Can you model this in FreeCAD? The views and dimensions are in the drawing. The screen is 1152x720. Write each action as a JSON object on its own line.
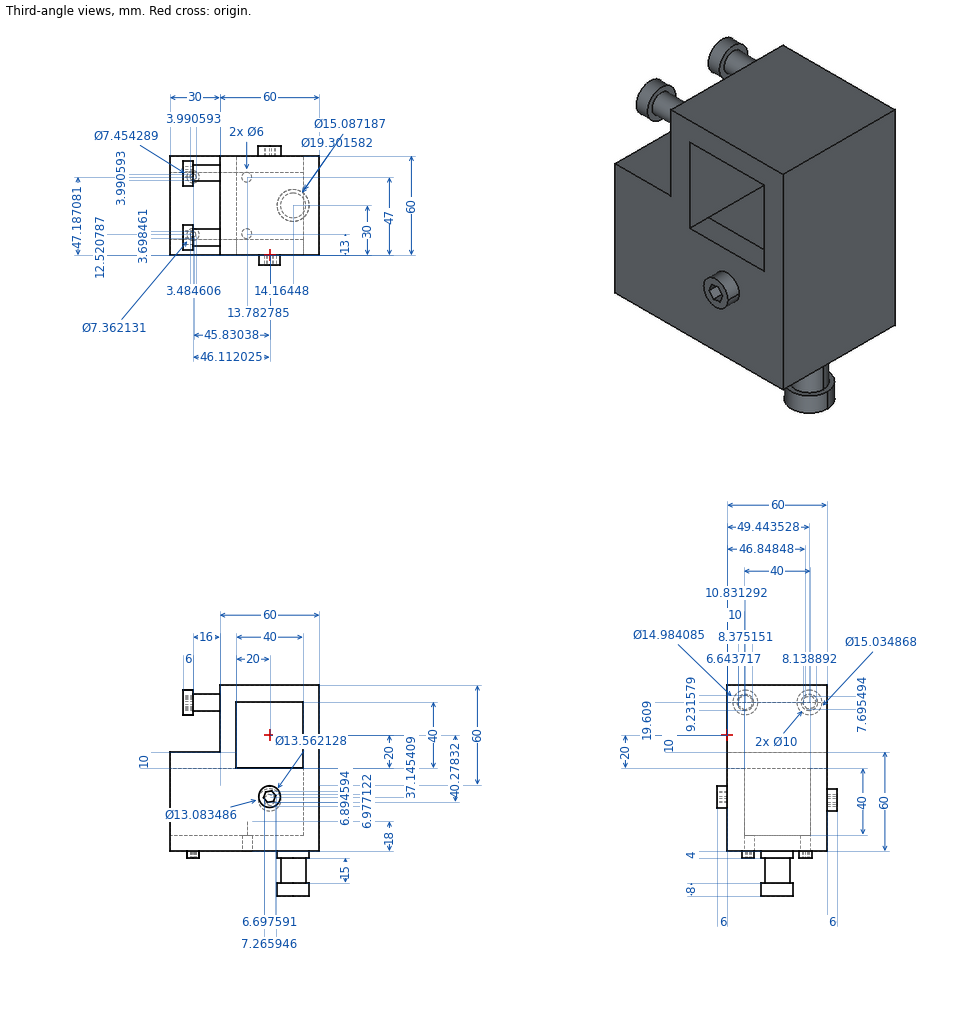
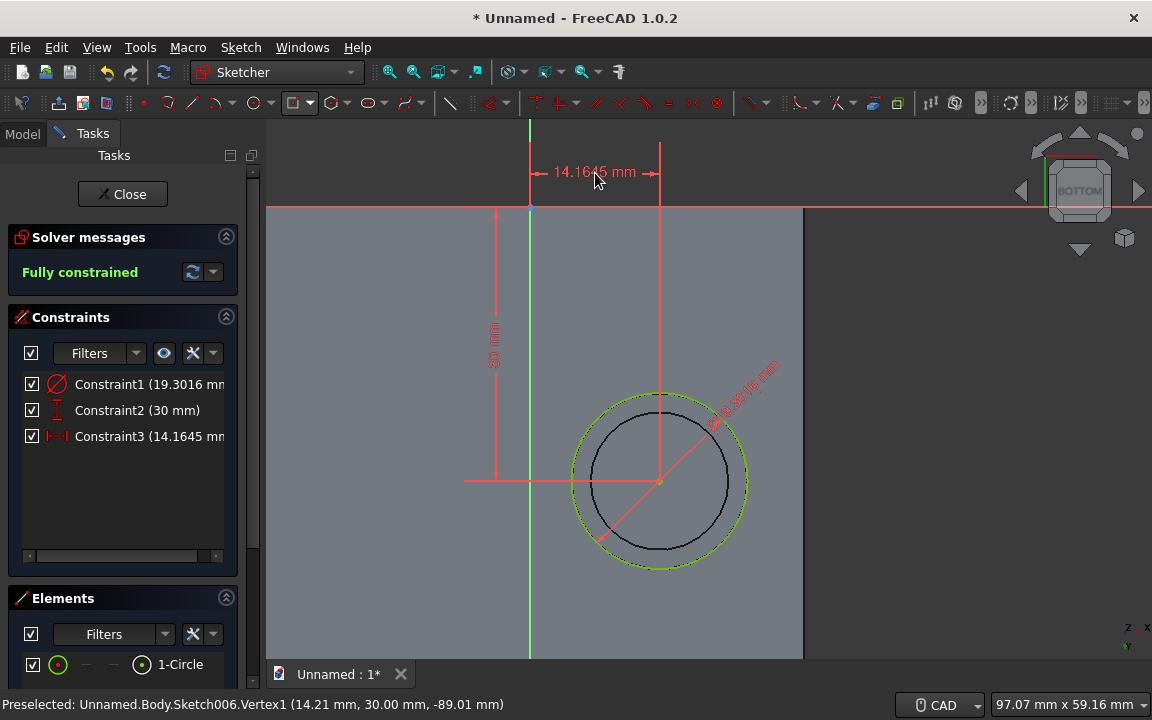
{"action": "left_click", "coordinate": [123, 194]}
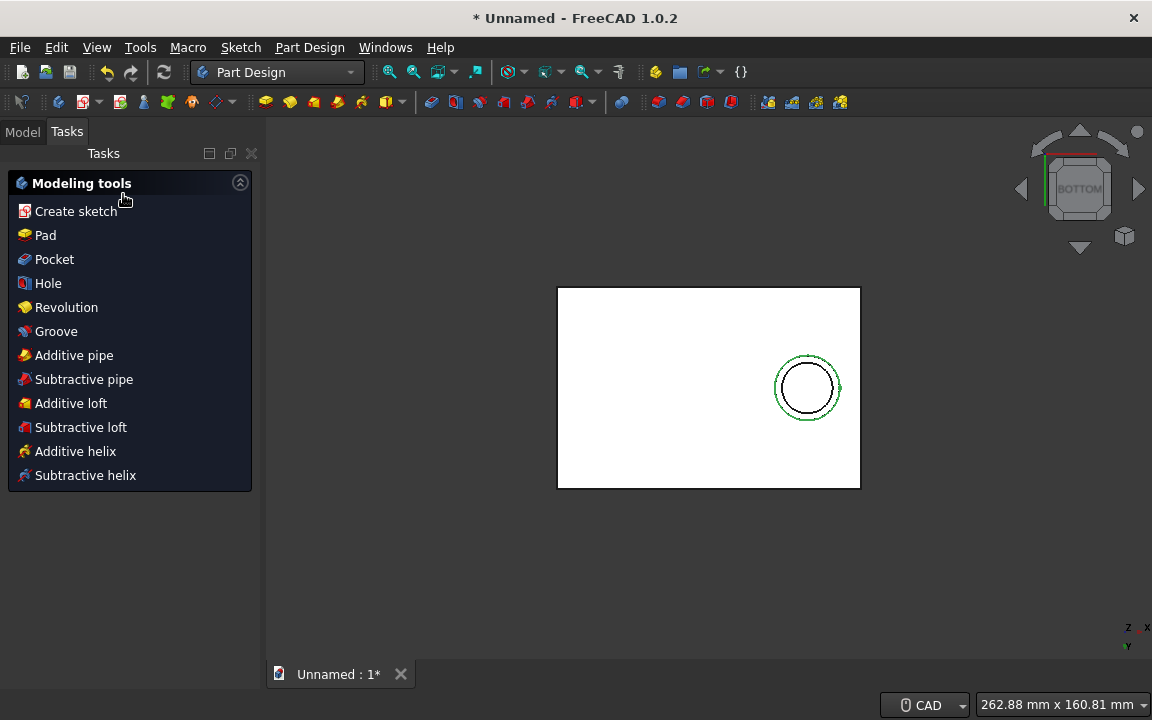
{"action": "left_click", "coordinate": [266, 102]}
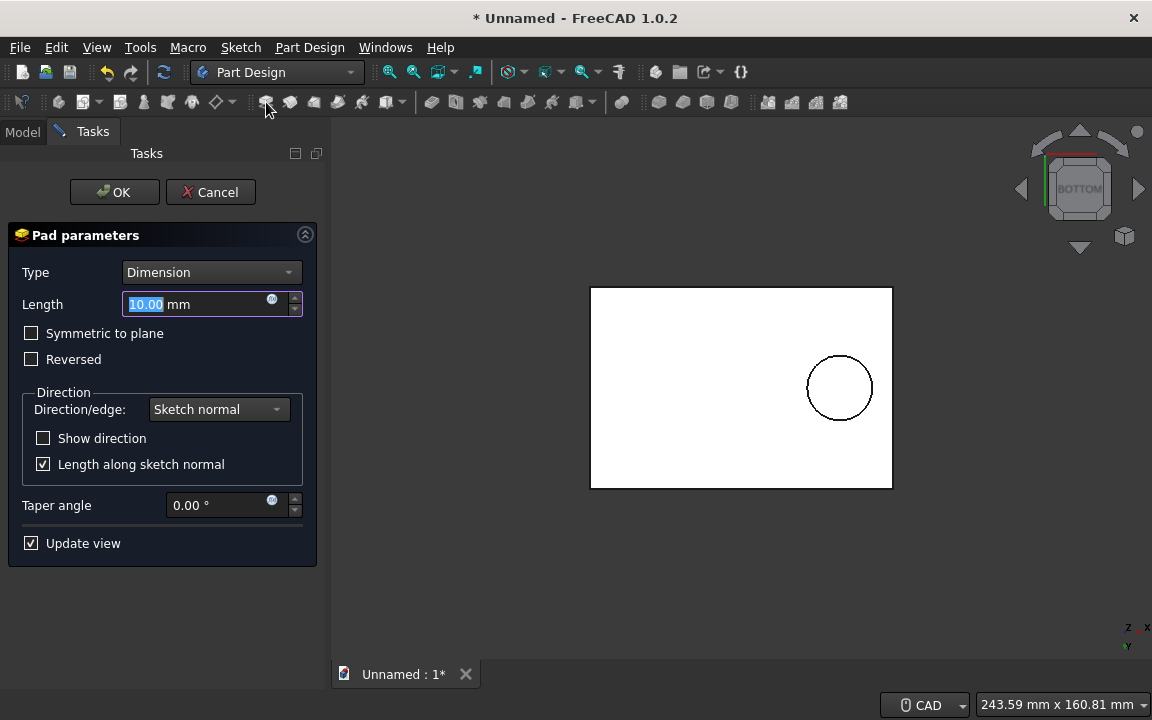
{"action": "type", "text": "8"}
{"action": "key", "text": "Tab"}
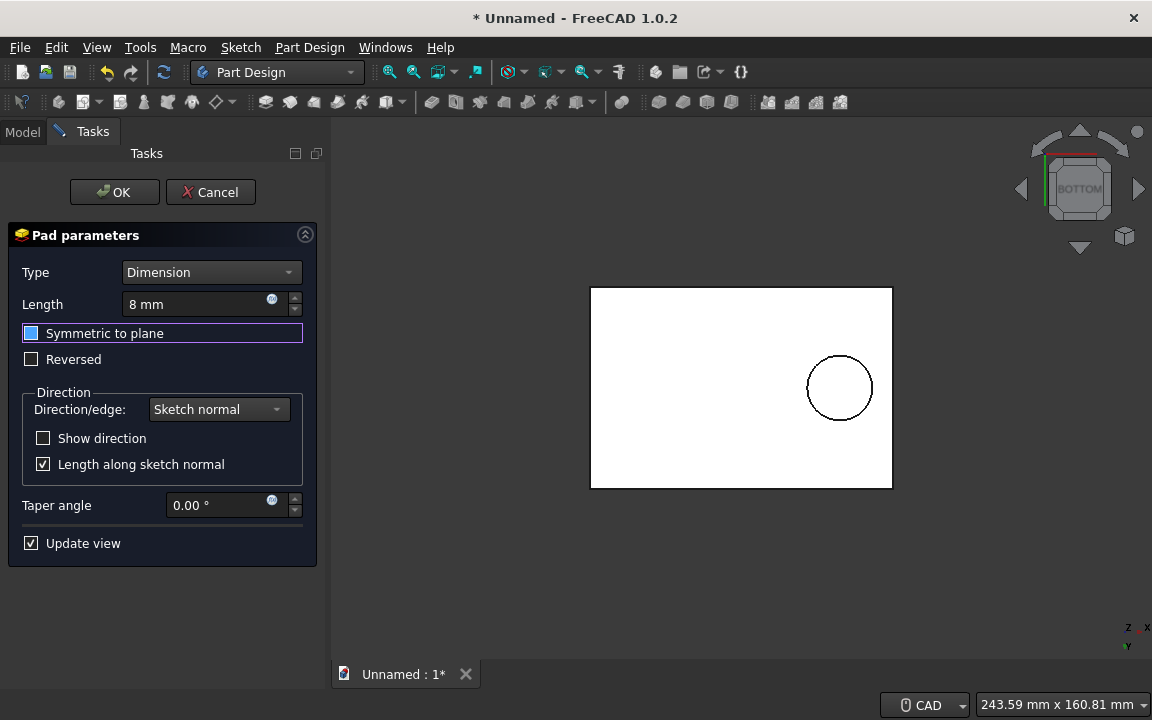
{"action": "left_click", "coordinate": [115, 192]}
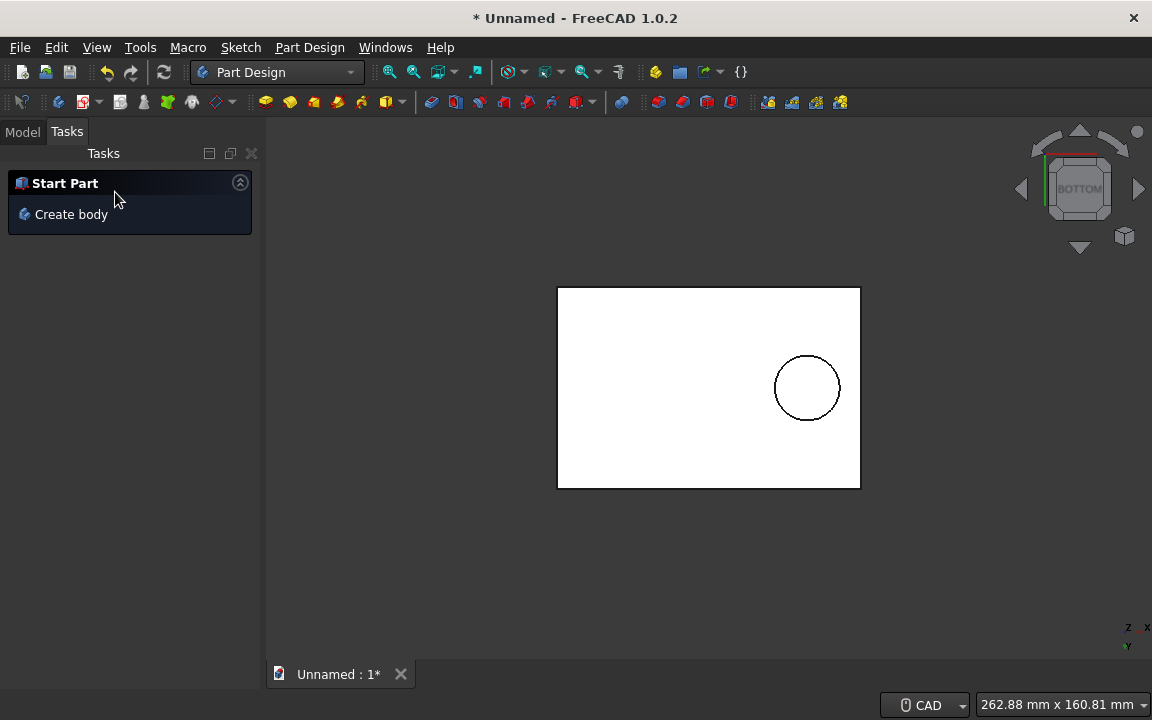
{"action": "left_click", "coordinate": [390, 72]}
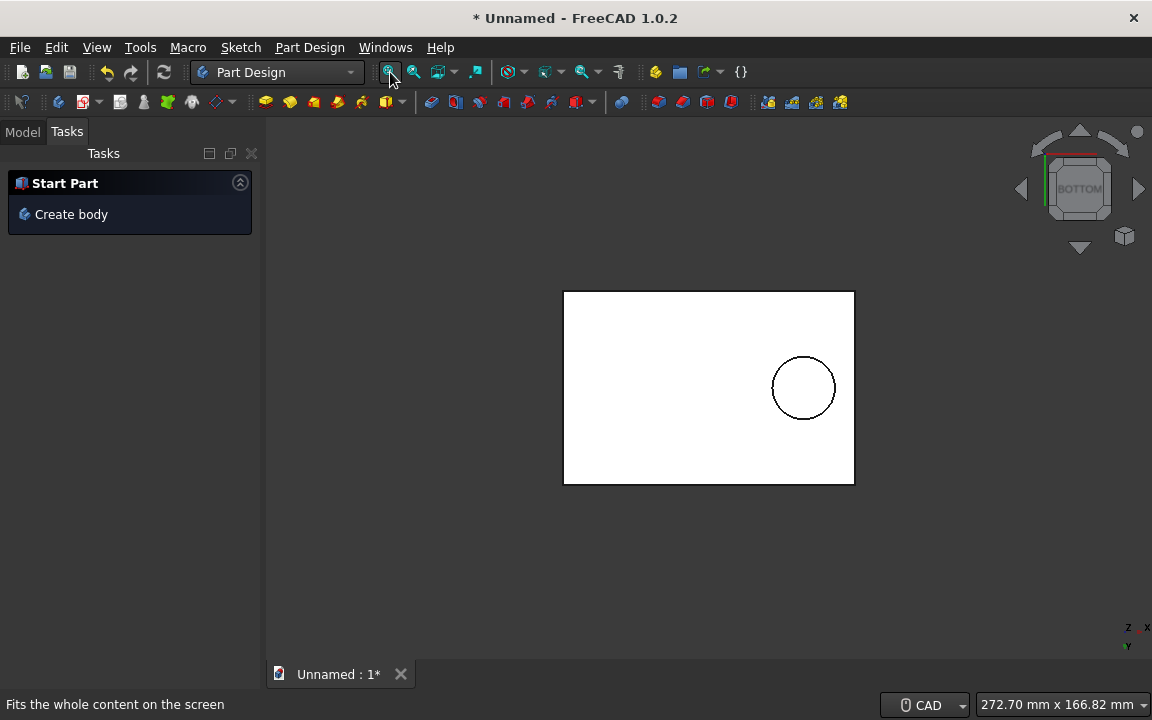
{"action": "left_click", "coordinate": [667, 387]}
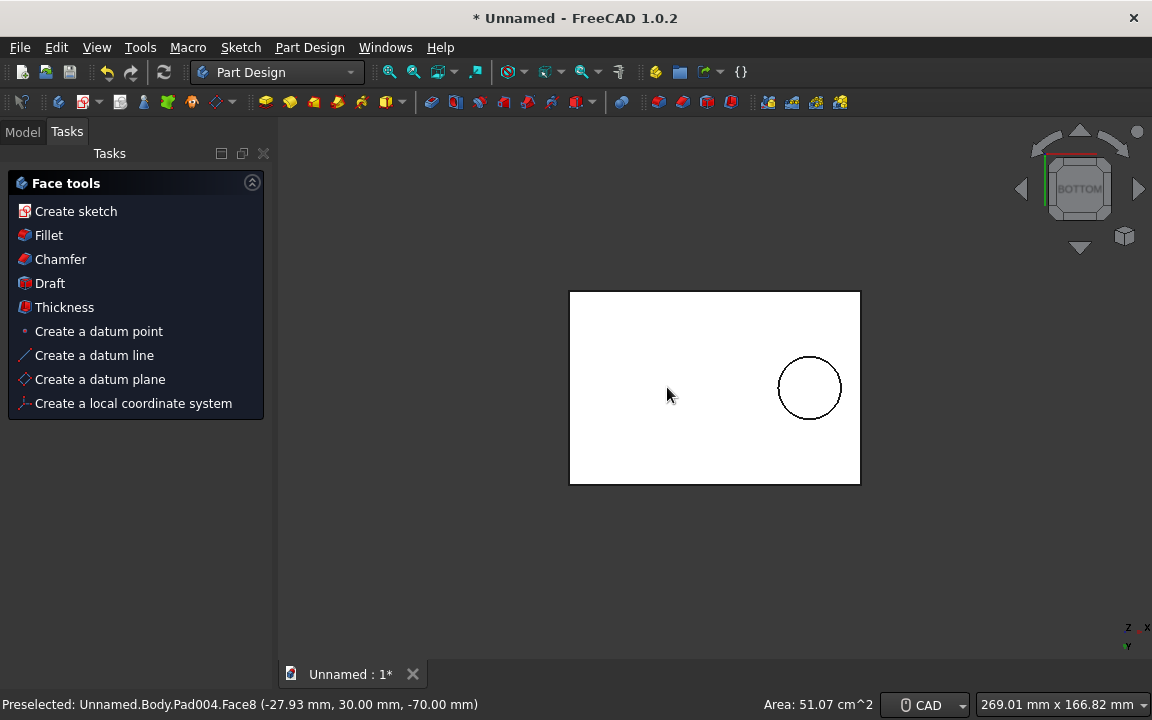
{"action": "left_click", "coordinate": [84, 102]}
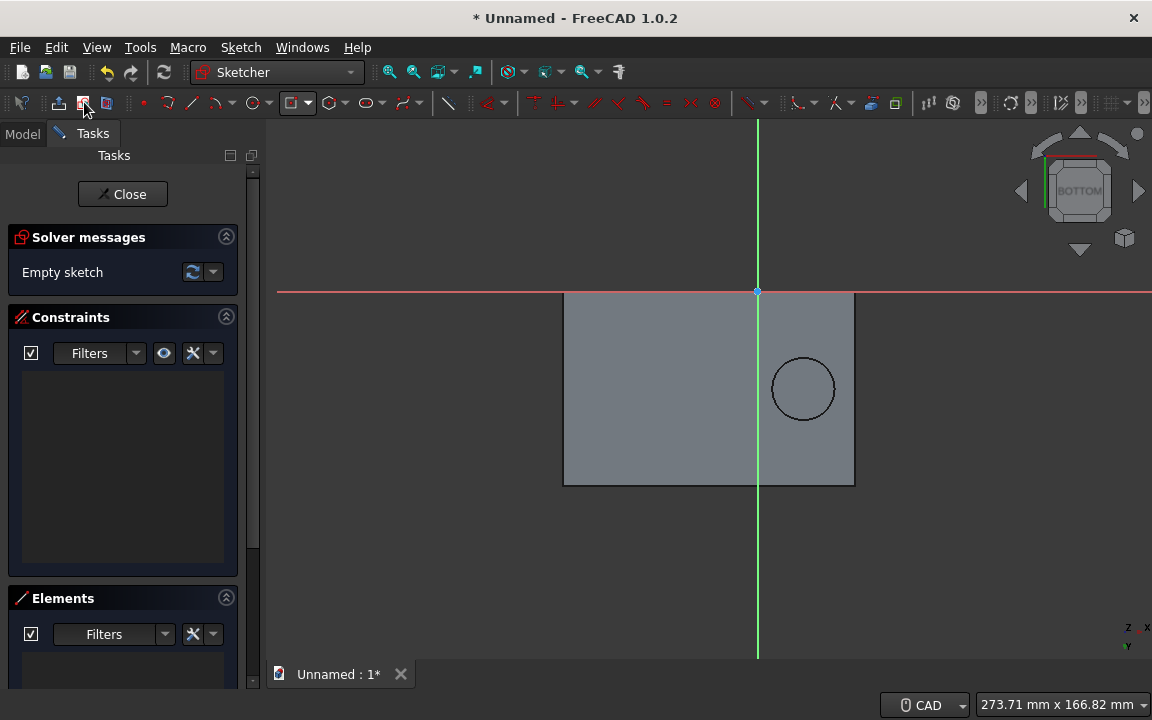
{"action": "scroll", "coordinate": [804, 360], "scroll_direction": "up", "scroll_amount": 4}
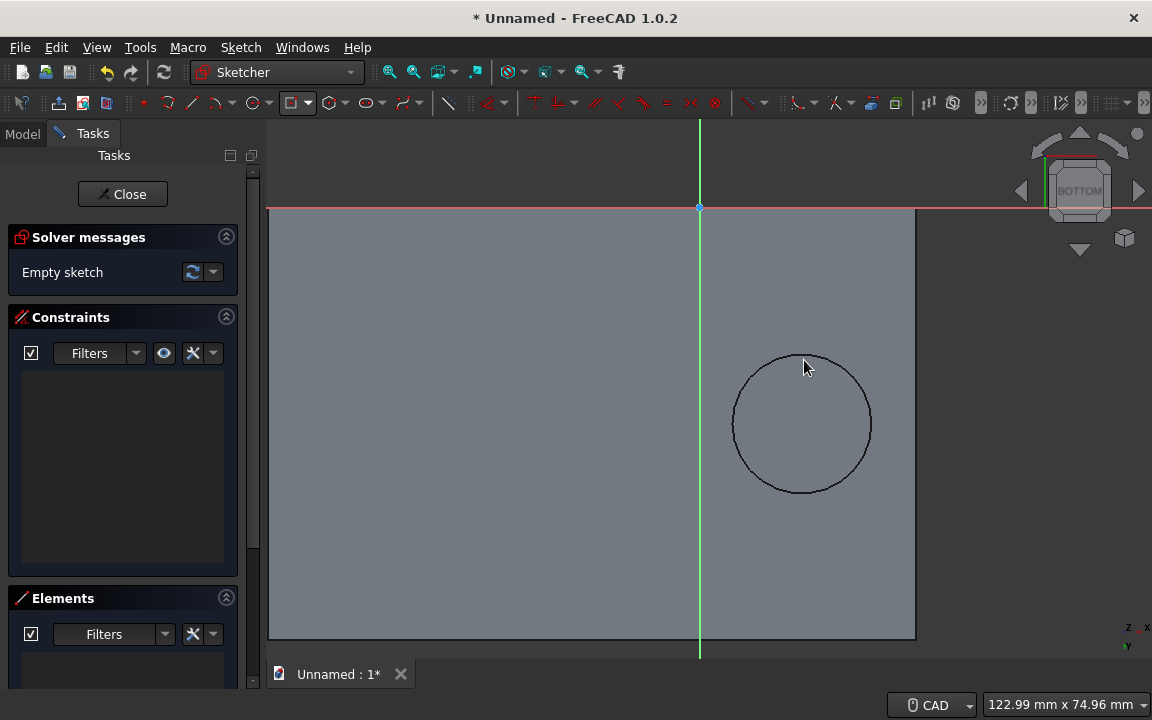
{"action": "left_click", "coordinate": [254, 104]}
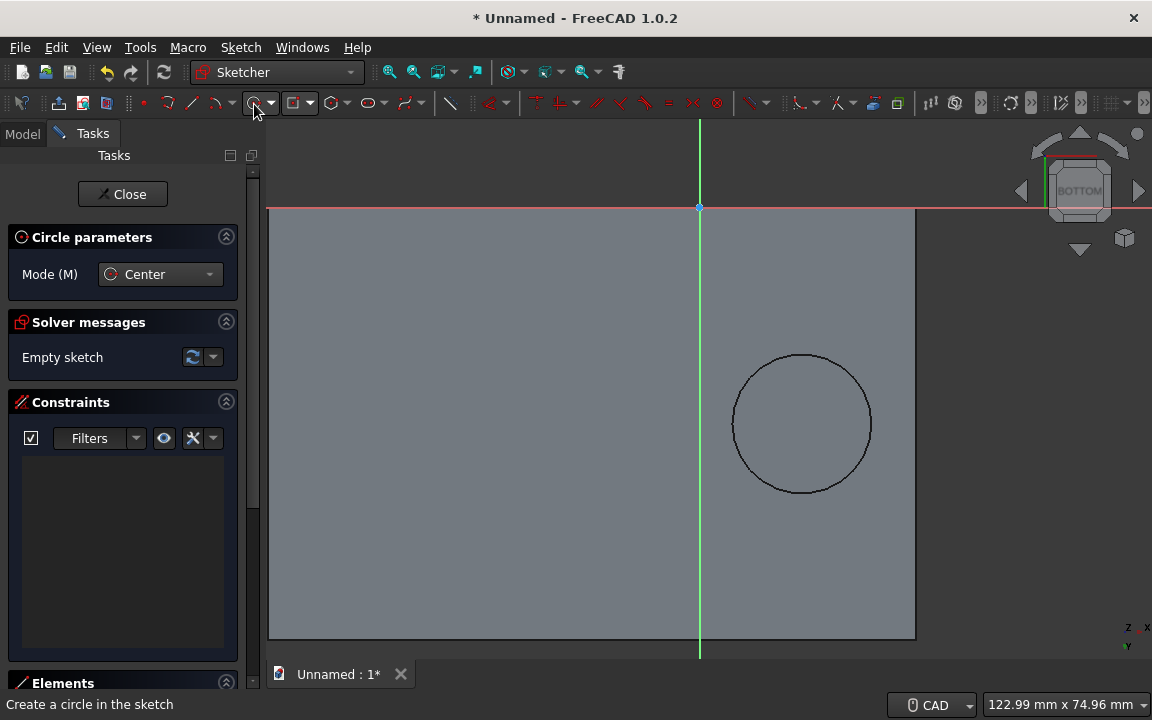
{"action": "left_click", "coordinate": [601, 546]}
{"action": "left_click", "coordinate": [616, 531]}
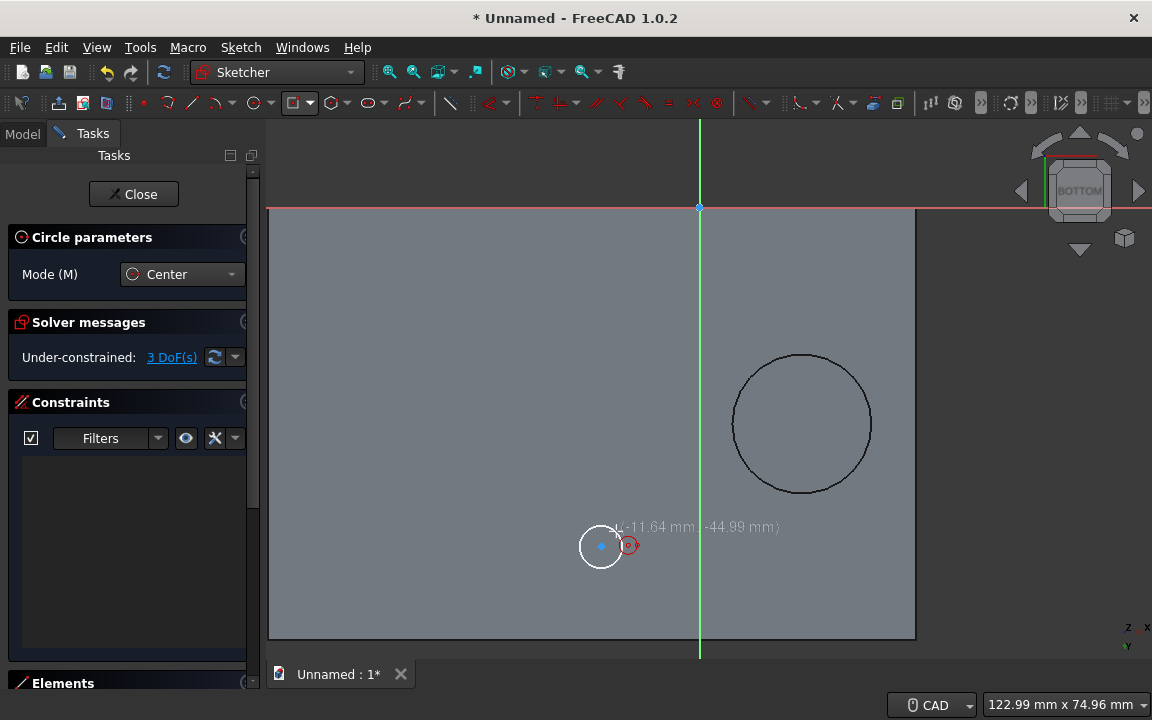
{"action": "left_click", "coordinate": [601, 302]}
{"action": "left_click", "coordinate": [616, 286]}
{"action": "key", "text": "Escape"}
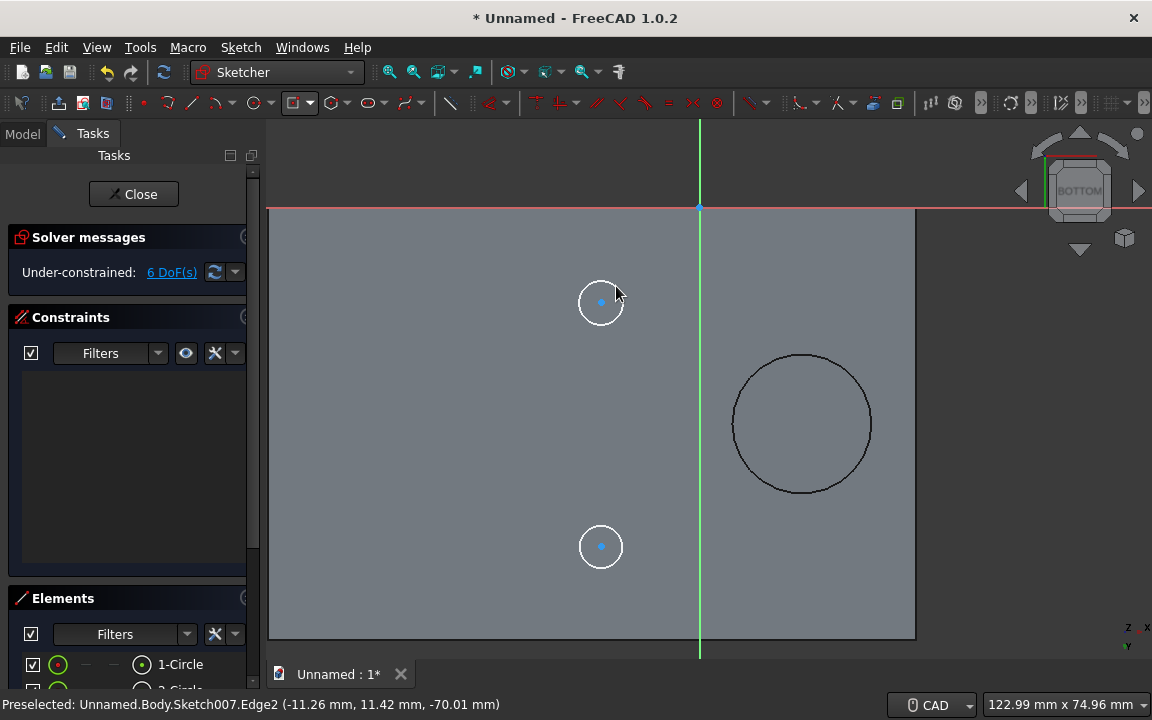
{"action": "left_click", "coordinate": [616, 532]}